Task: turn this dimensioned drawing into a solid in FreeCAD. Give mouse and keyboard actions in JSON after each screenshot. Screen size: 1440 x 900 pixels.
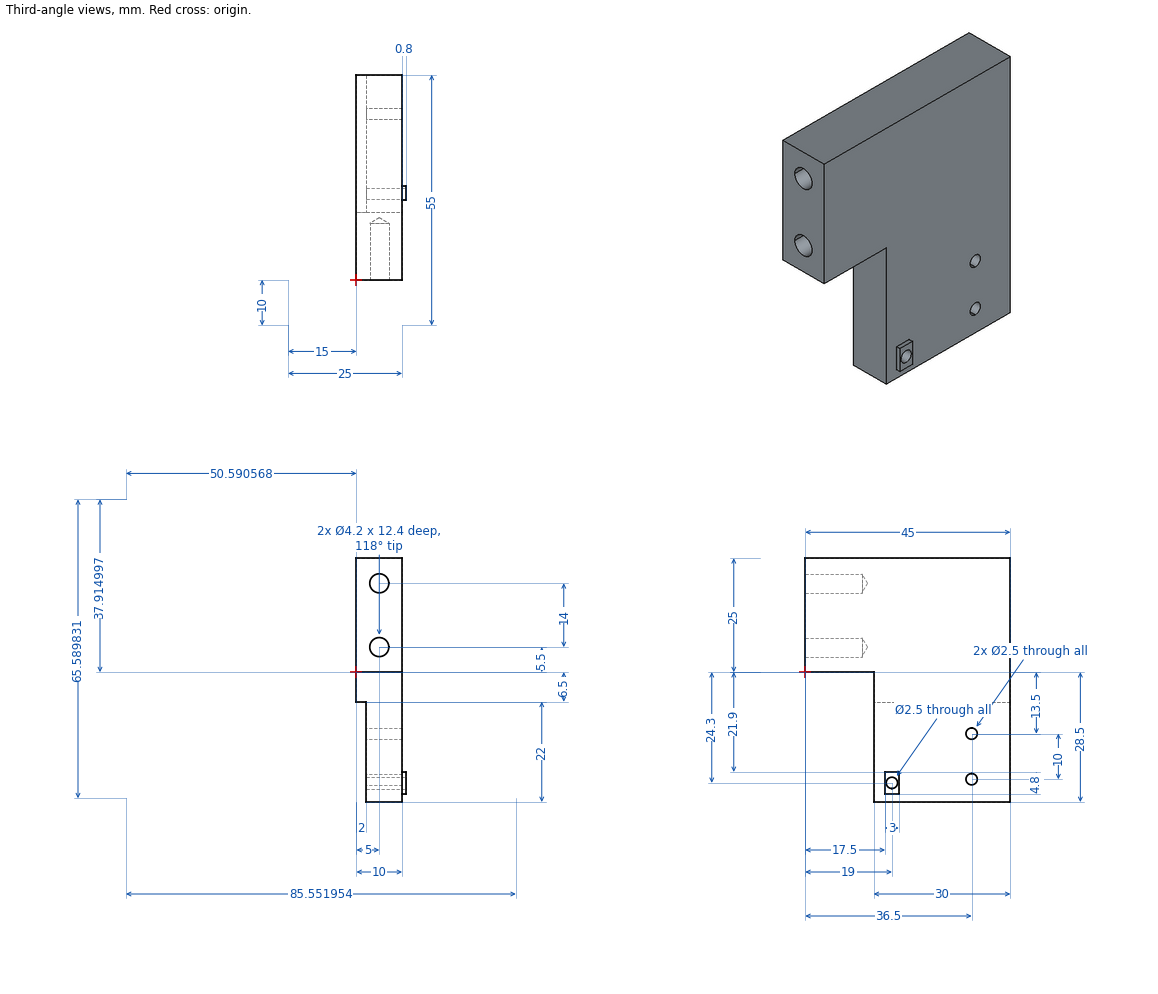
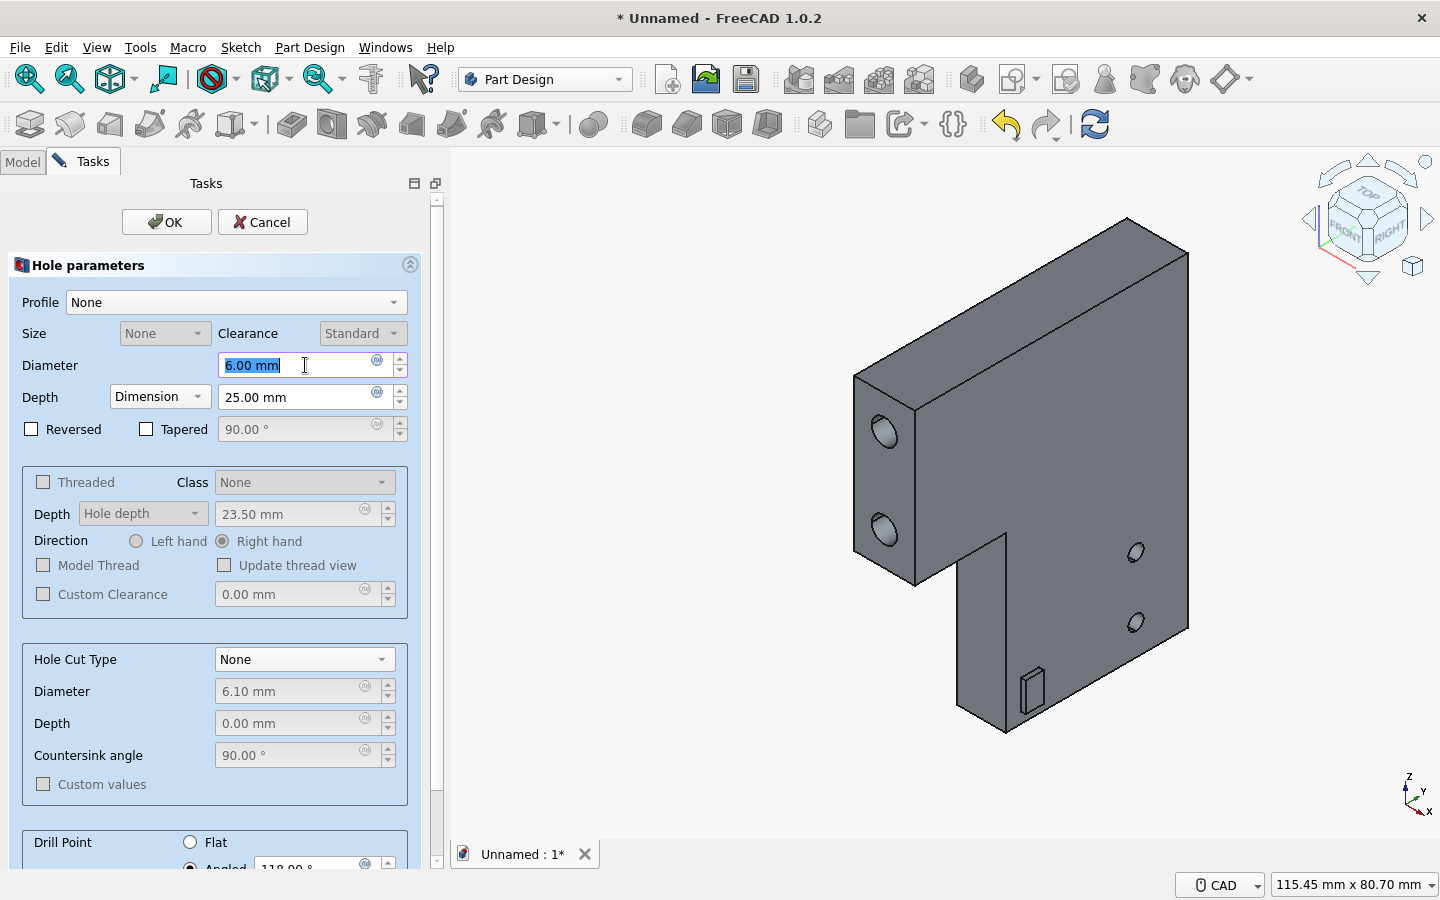
{"action": "type", "text": "2.5"}
{"action": "key", "text": "Tab"}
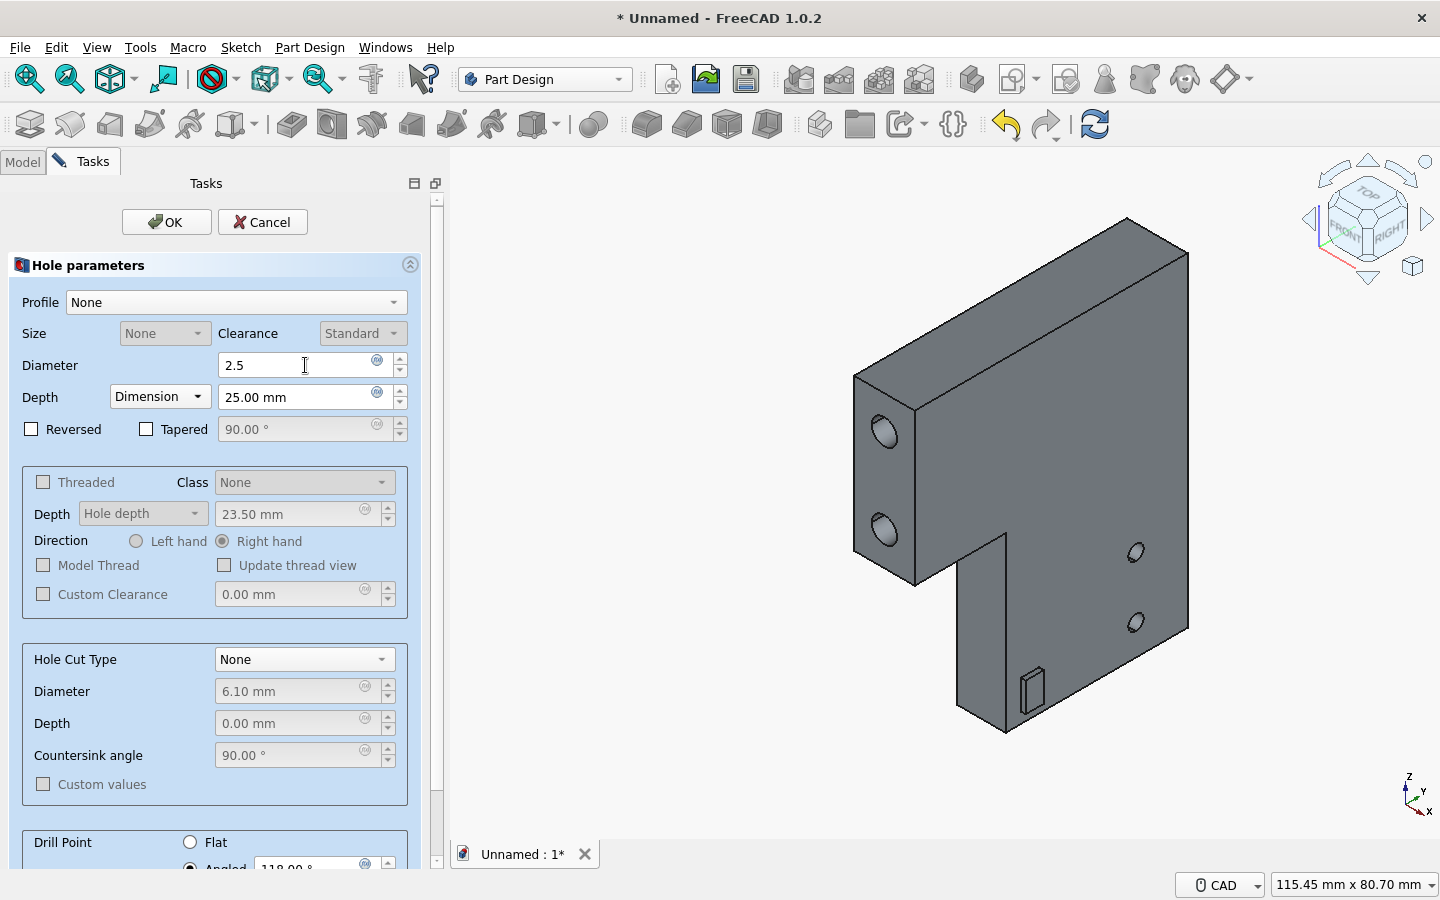
{"action": "left_click", "coordinate": [161, 396]}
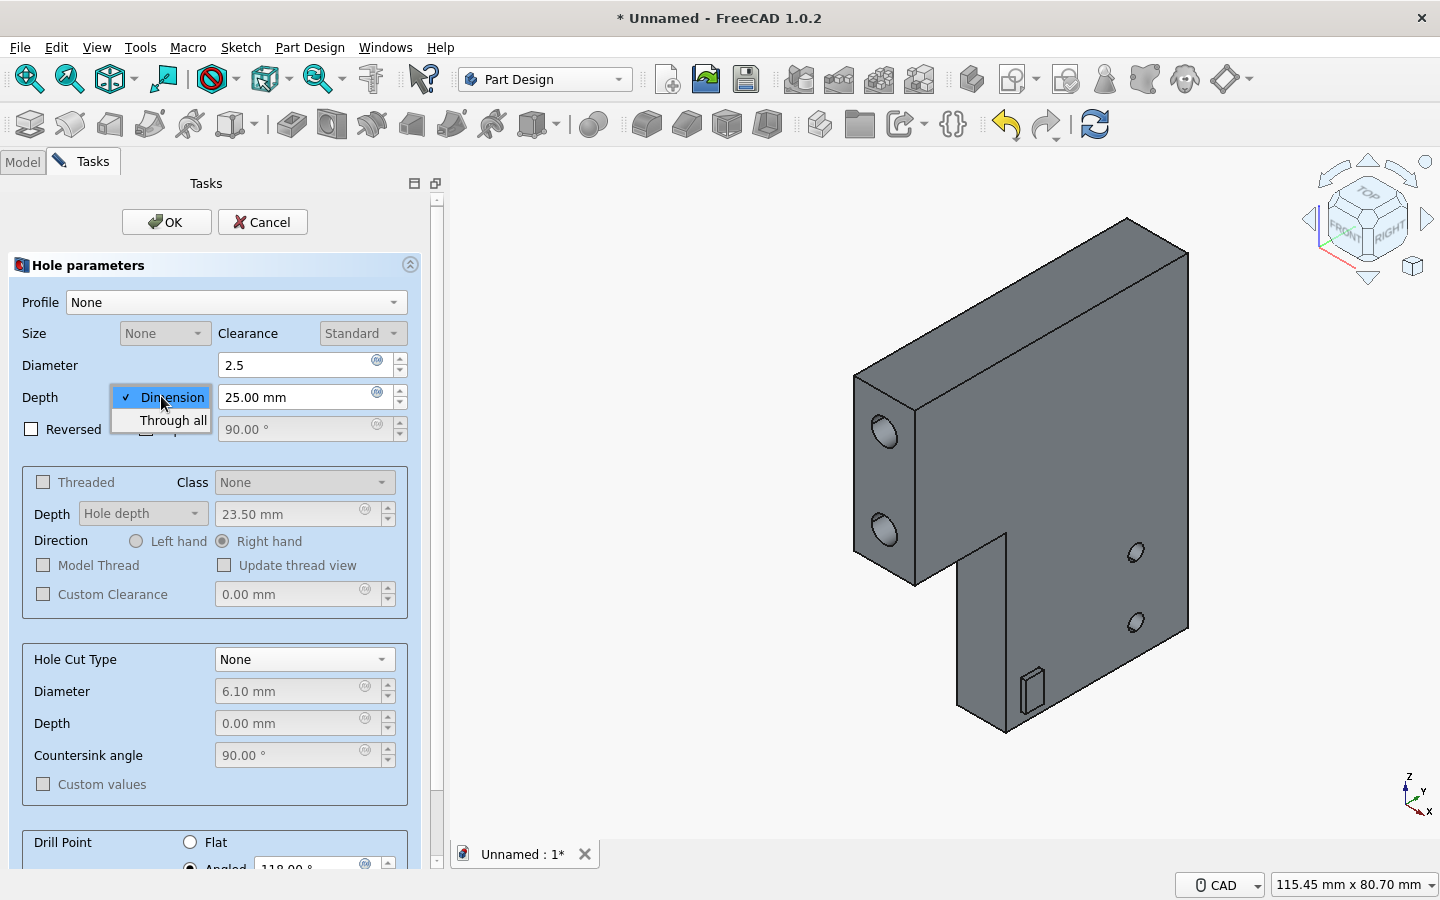
{"action": "left_click", "coordinate": [160, 420]}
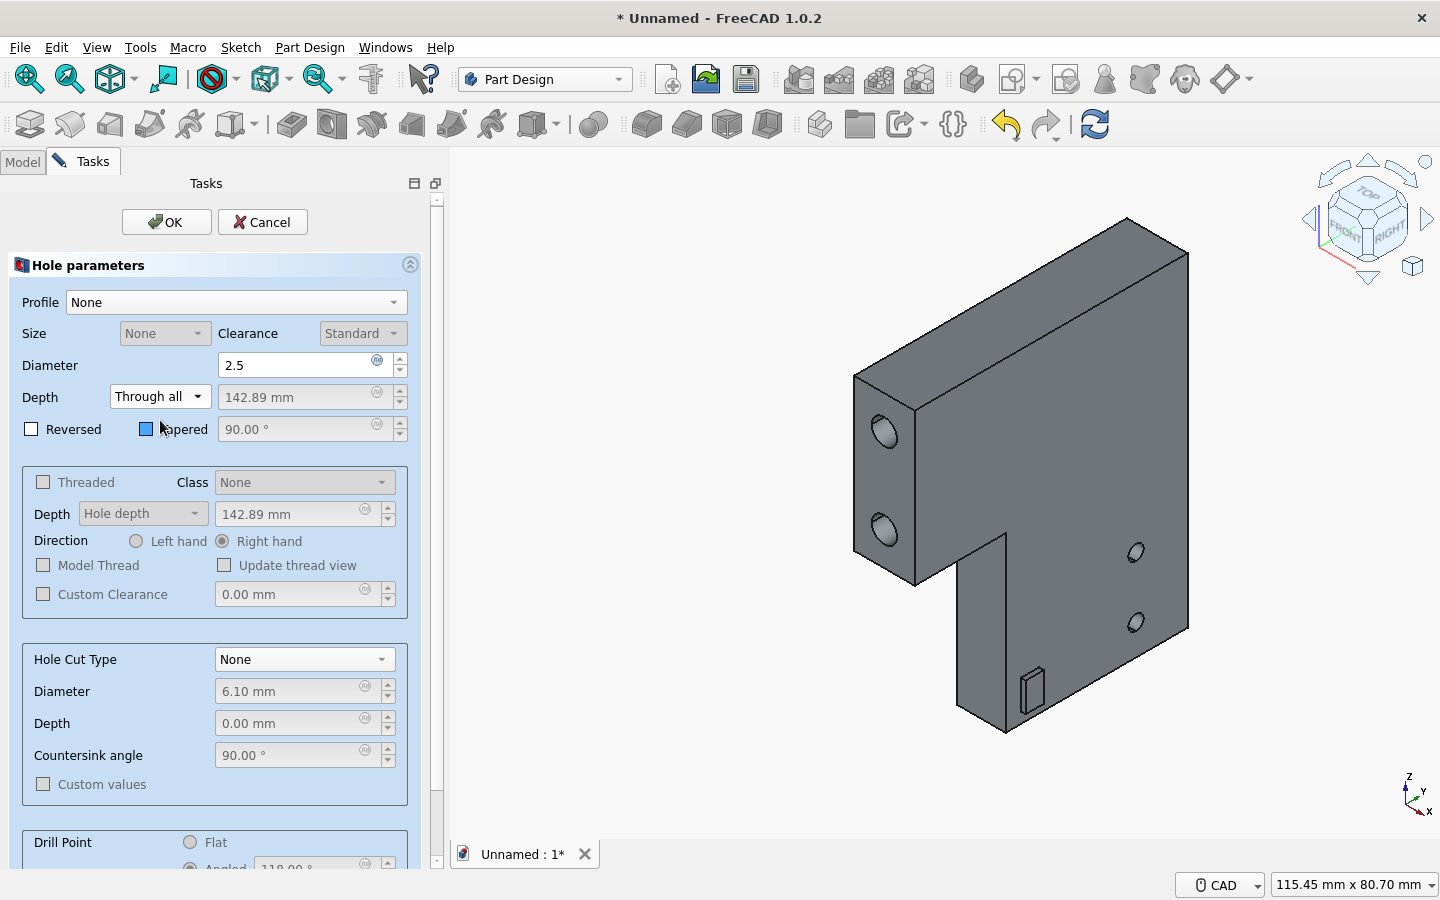
{"action": "left_click", "coordinate": [30, 429]}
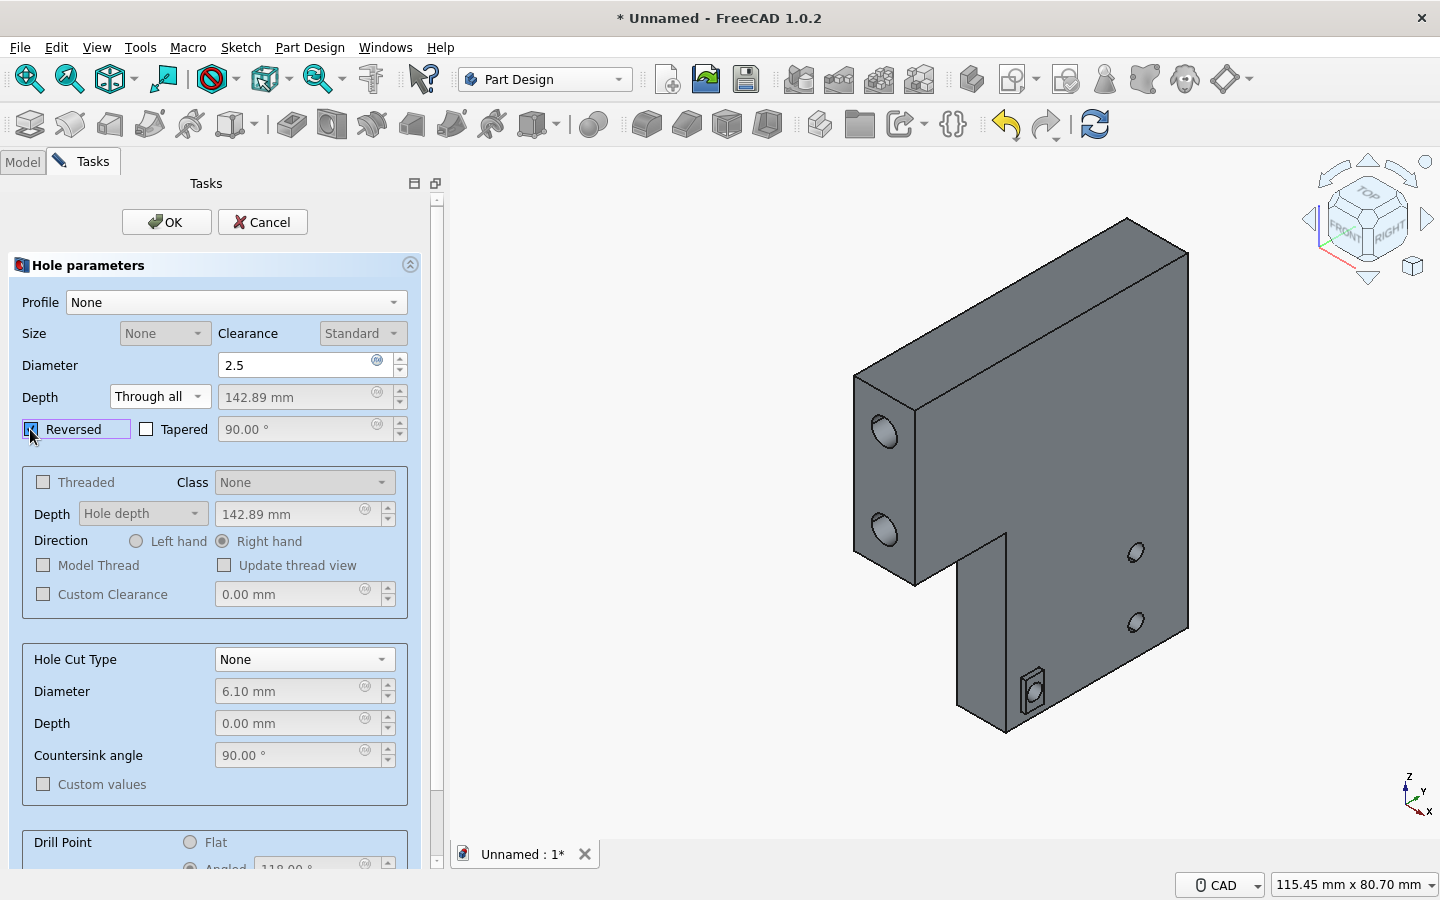
{"action": "left_click", "coordinate": [167, 222]}